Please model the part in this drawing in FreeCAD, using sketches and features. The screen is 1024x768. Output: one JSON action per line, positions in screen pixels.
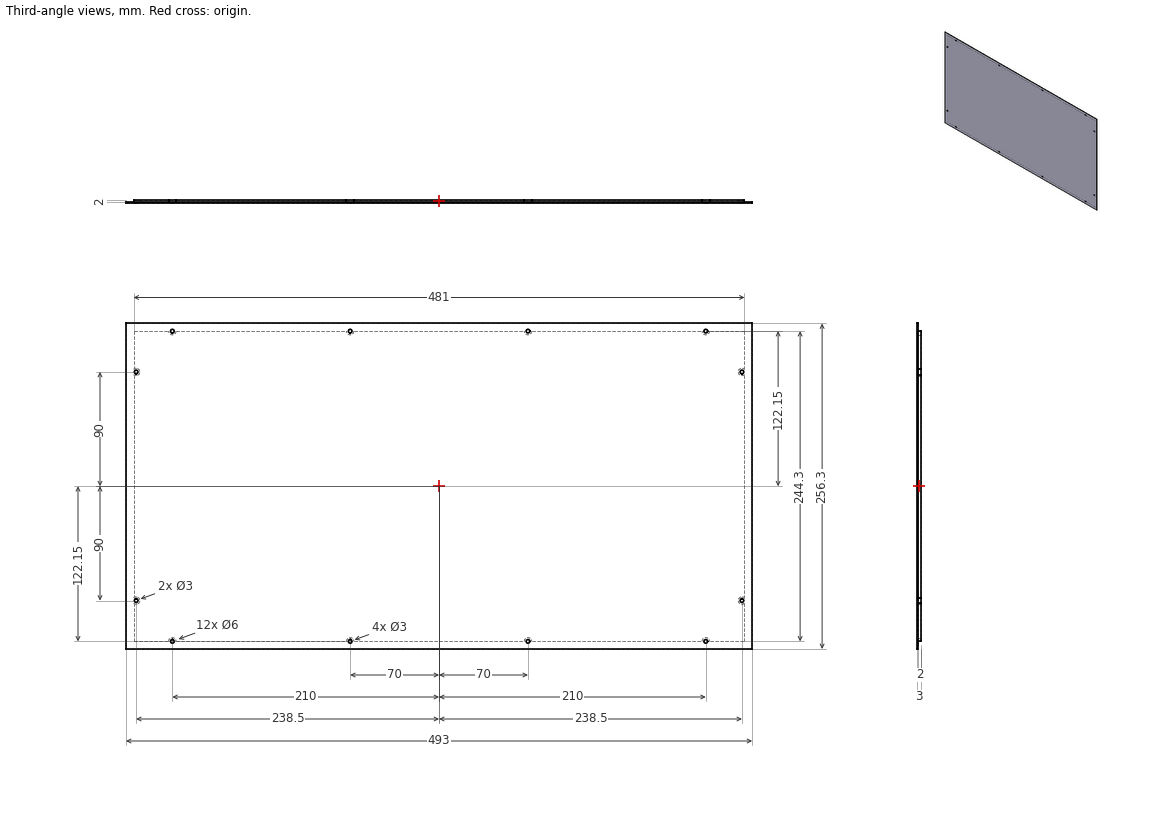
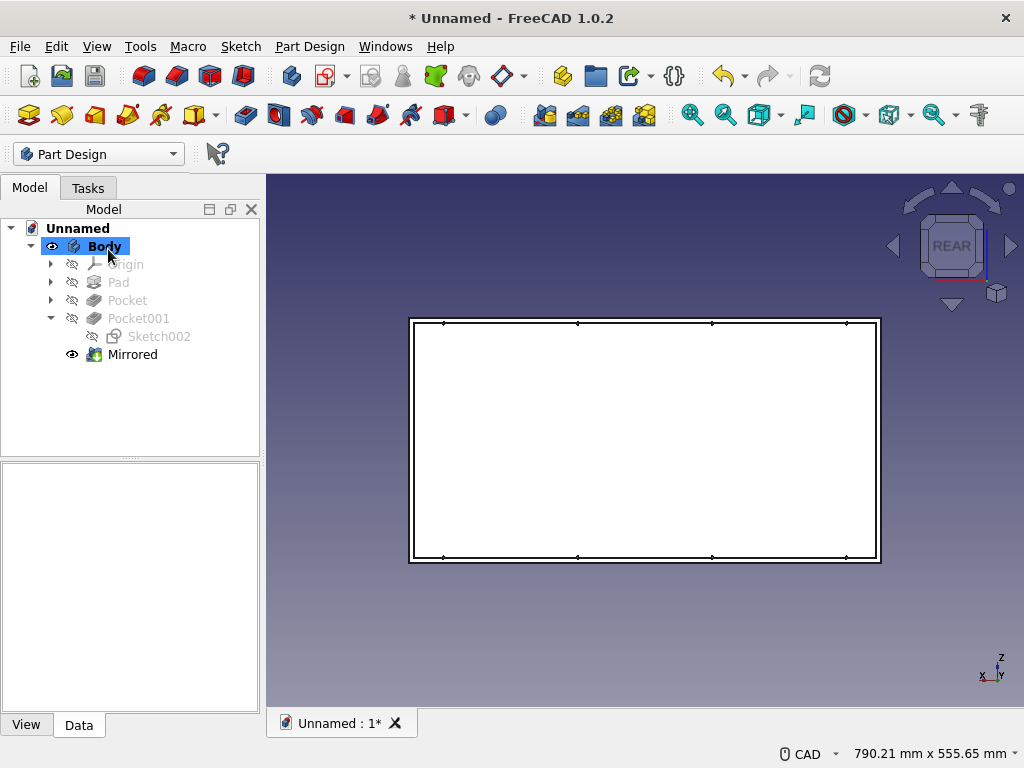
{"action": "left_click", "coordinate": [645, 440]}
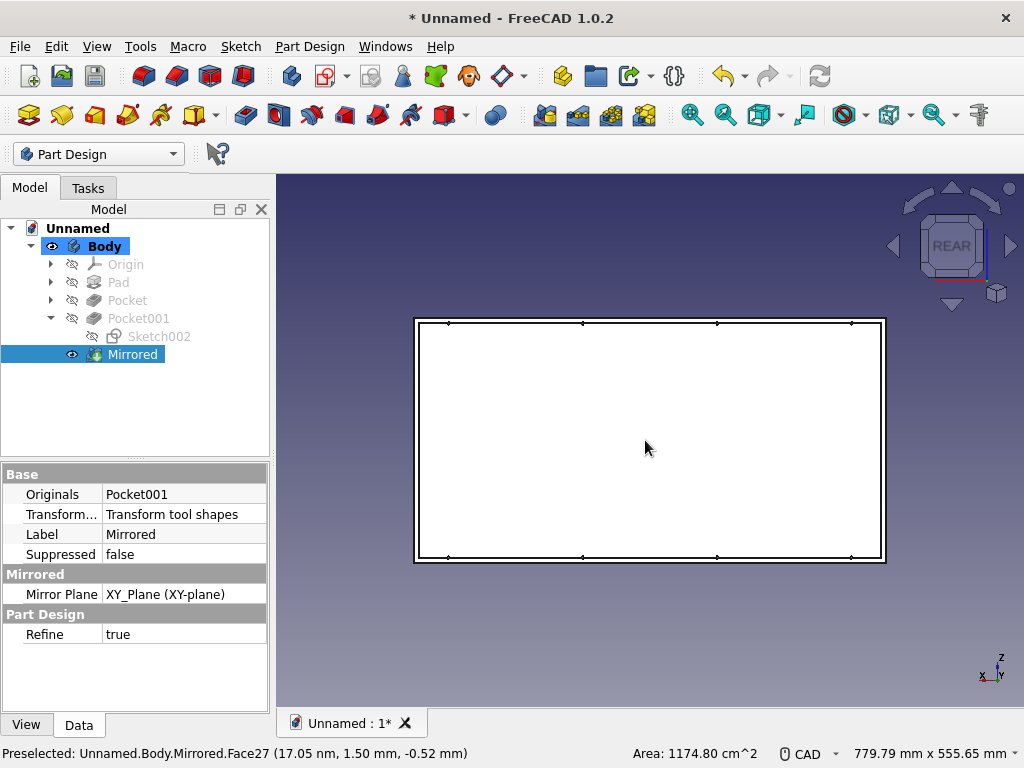
{"action": "left_click", "coordinate": [324, 76]}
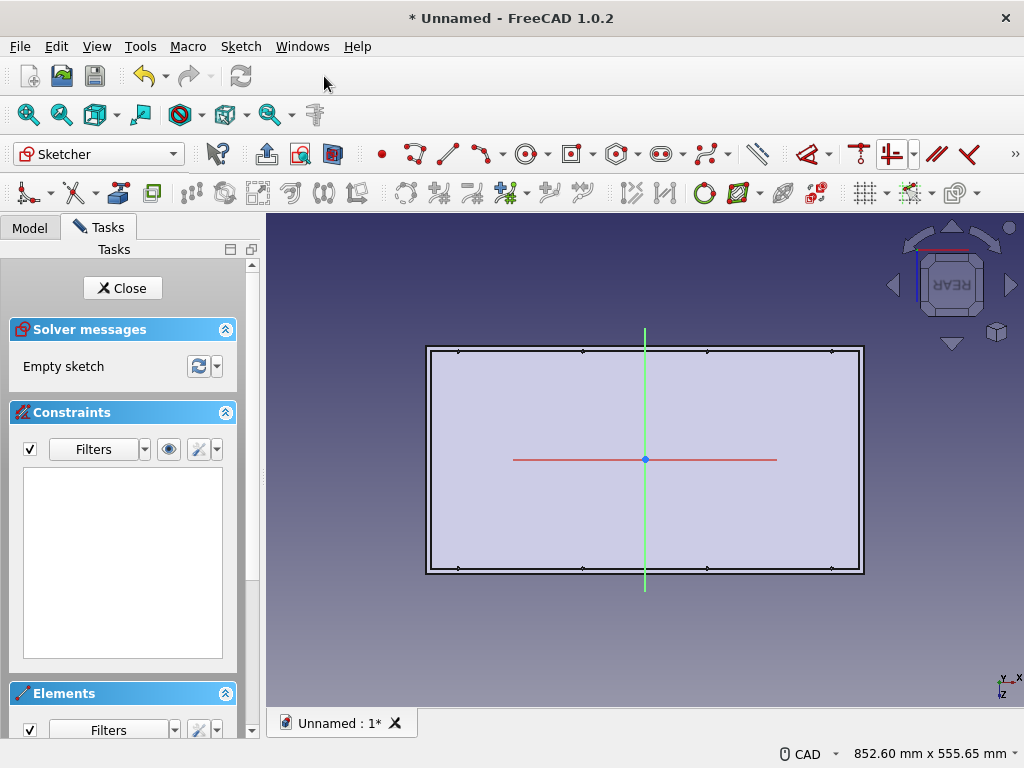
{"action": "scroll", "coordinate": [492, 460], "scroll_direction": "up", "scroll_amount": 3}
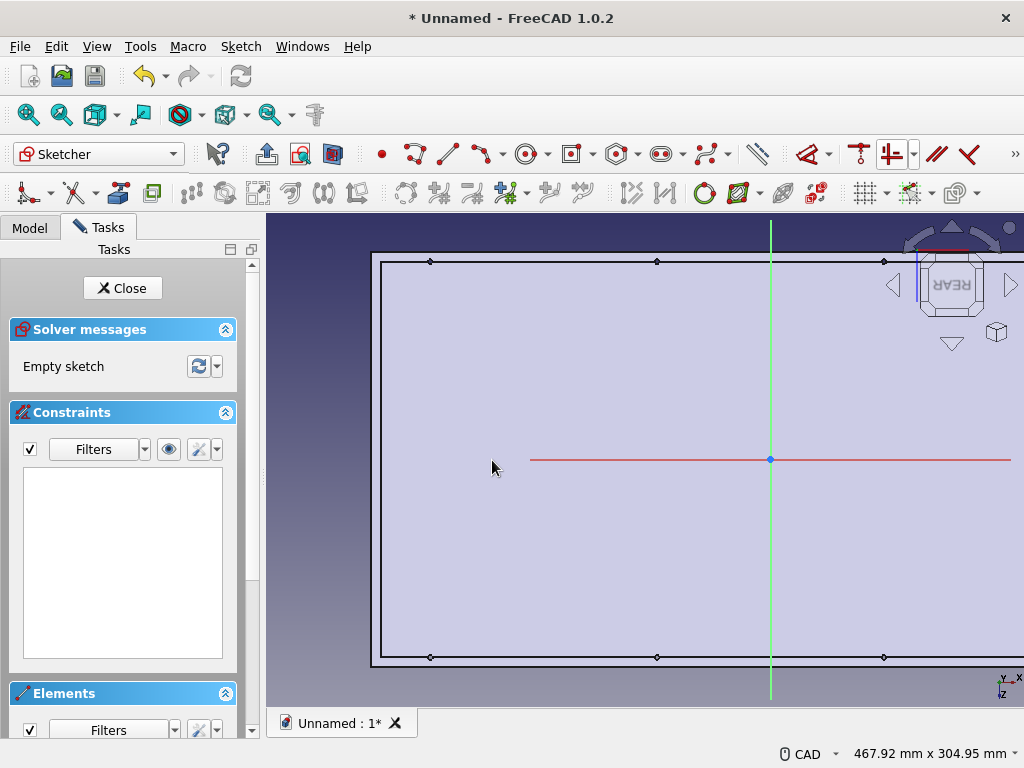
{"action": "left_click", "coordinate": [526, 154]}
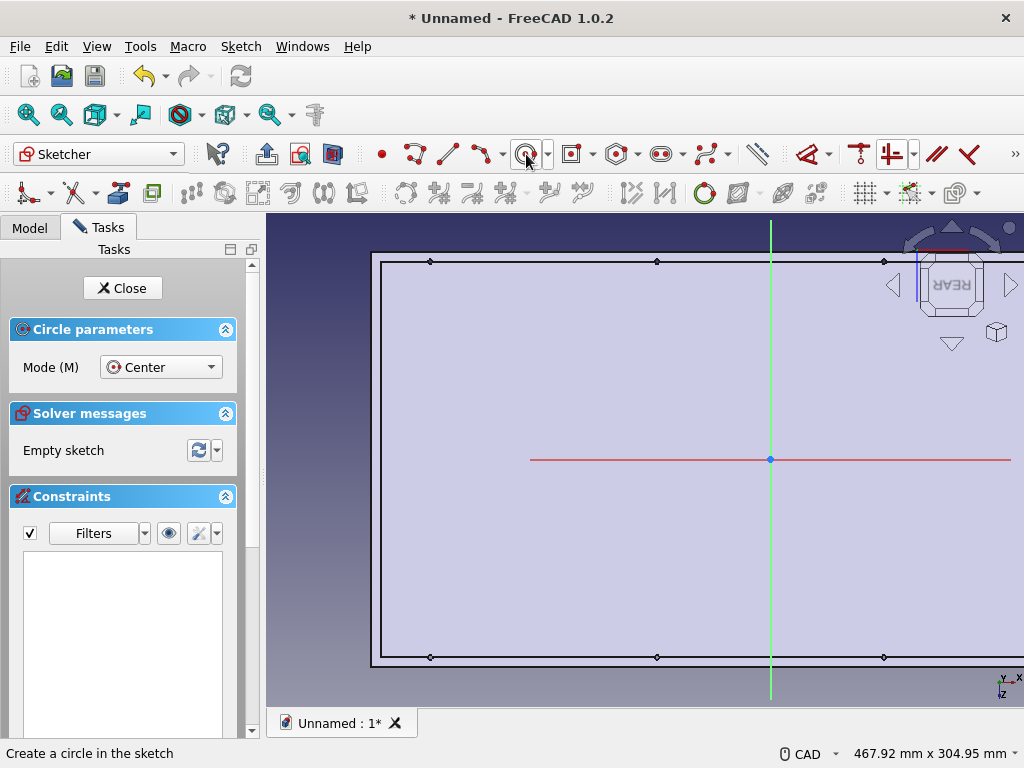
{"action": "scroll", "coordinate": [384, 314], "scroll_direction": "up", "scroll_amount": 12}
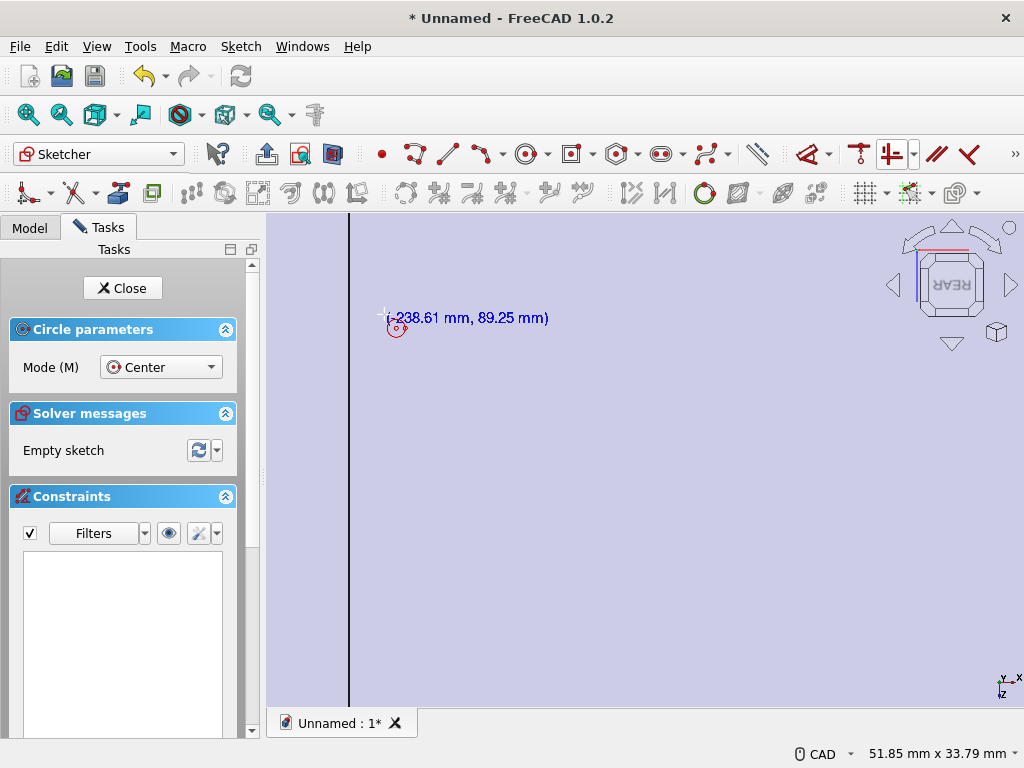
{"action": "scroll", "coordinate": [385, 315], "scroll_direction": "down", "scroll_amount": 12}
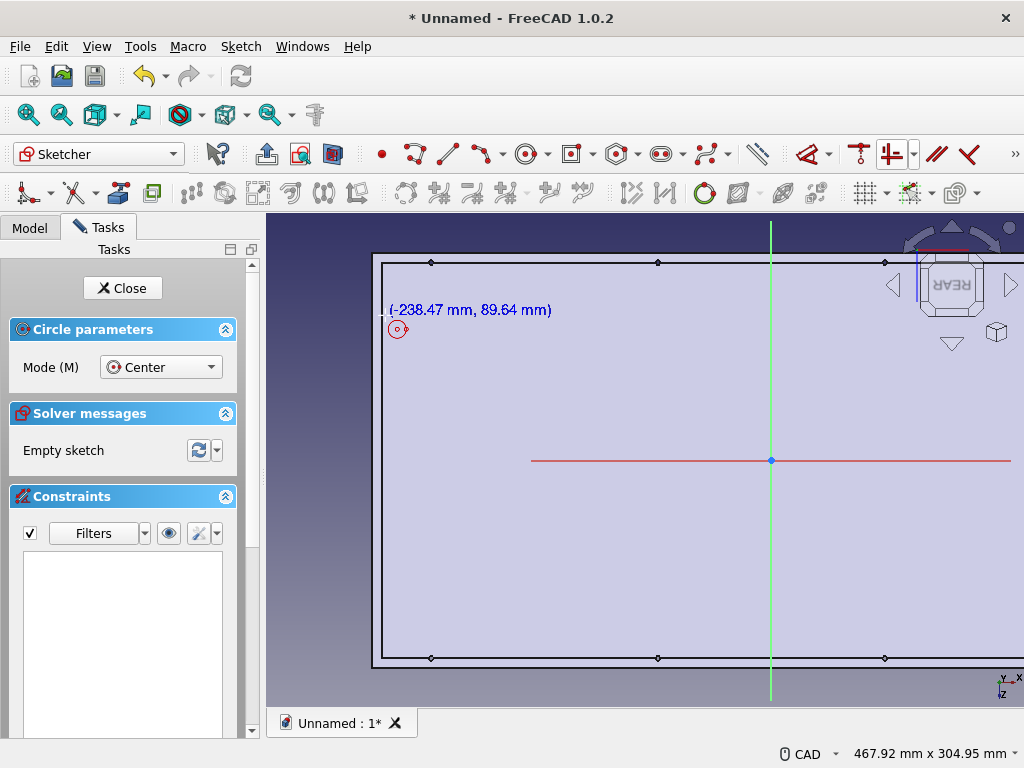
{"action": "left_click", "coordinate": [385, 315]}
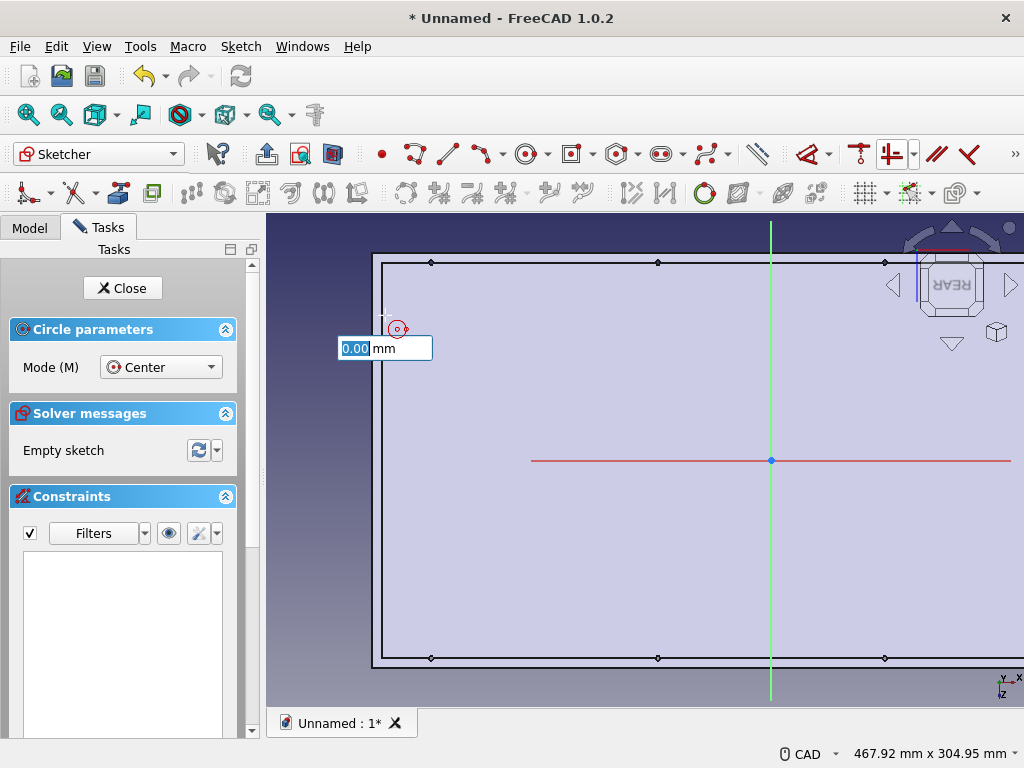
{"action": "scroll", "coordinate": [387, 313], "scroll_direction": "up", "scroll_amount": 10}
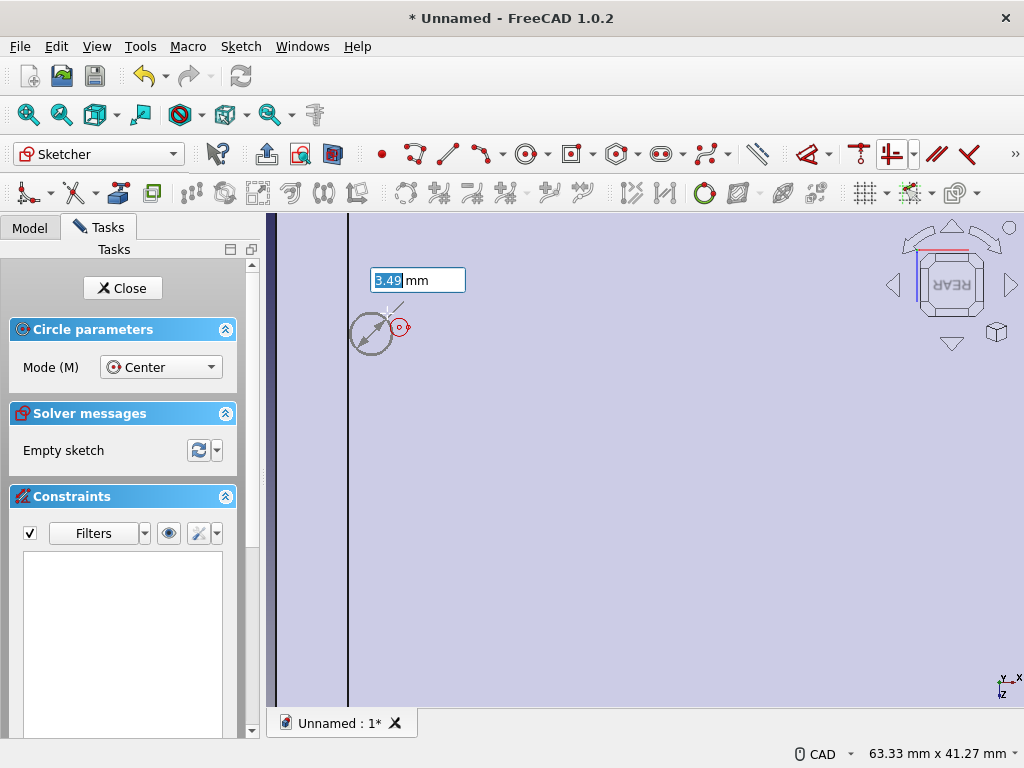
{"action": "left_click", "coordinate": [385, 312]}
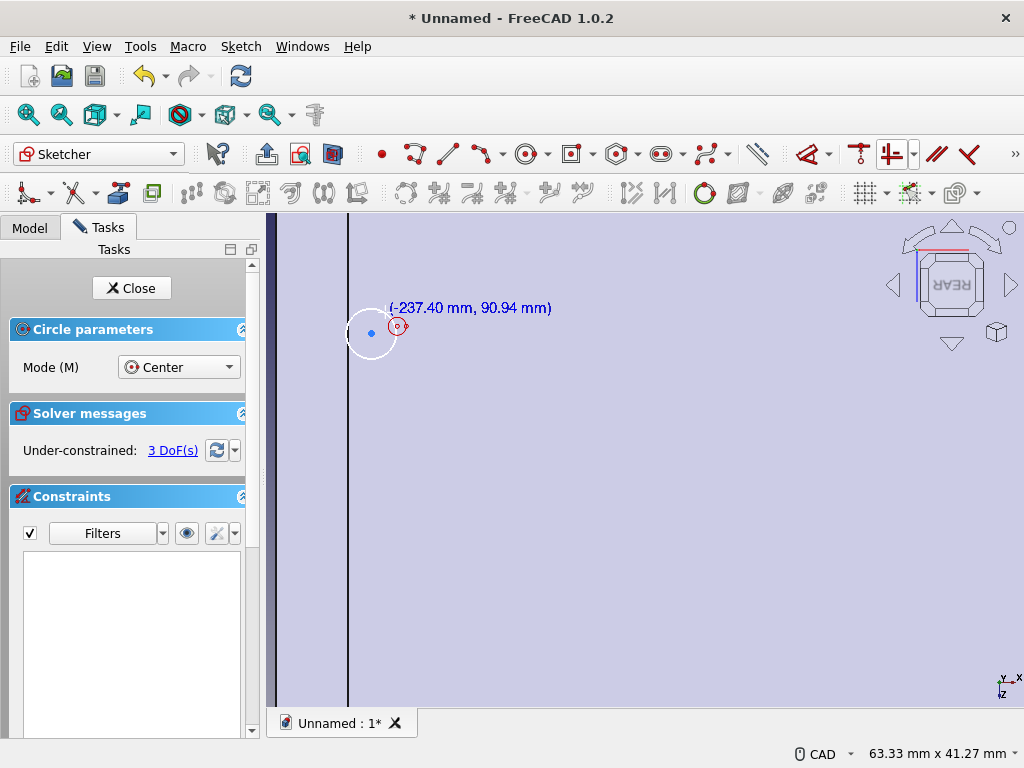
{"action": "scroll", "coordinate": [387, 313], "scroll_direction": "down", "scroll_amount": 10}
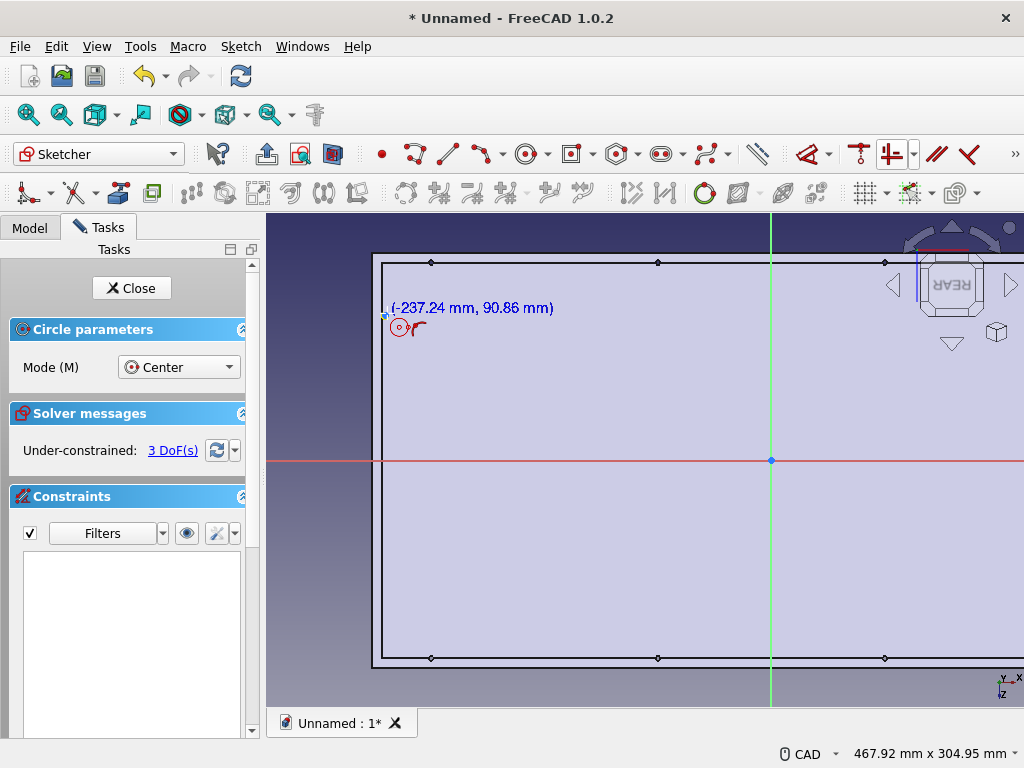
{"action": "scroll", "coordinate": [385, 606], "scroll_direction": "up", "scroll_amount": 12}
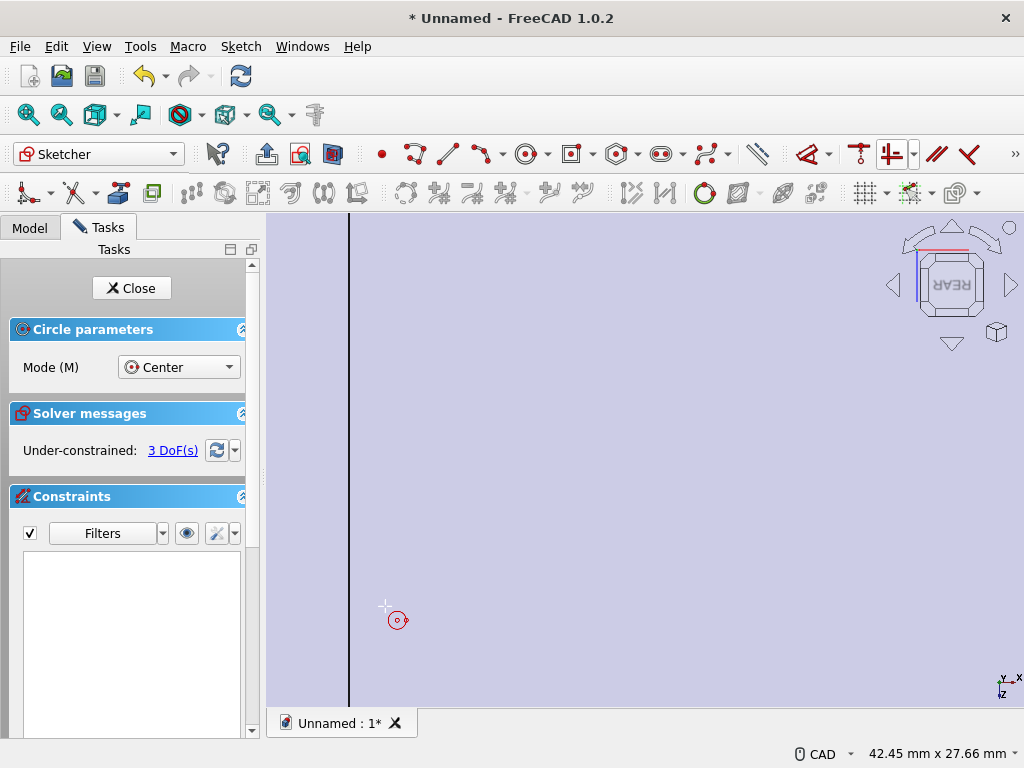
{"action": "scroll", "coordinate": [385, 606], "scroll_direction": "down", "scroll_amount": 12}